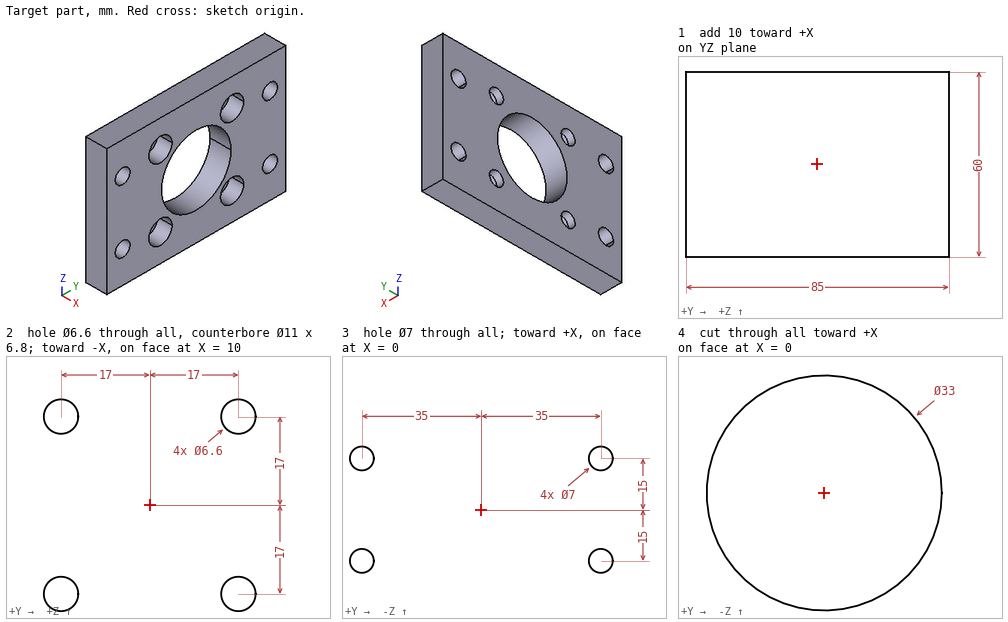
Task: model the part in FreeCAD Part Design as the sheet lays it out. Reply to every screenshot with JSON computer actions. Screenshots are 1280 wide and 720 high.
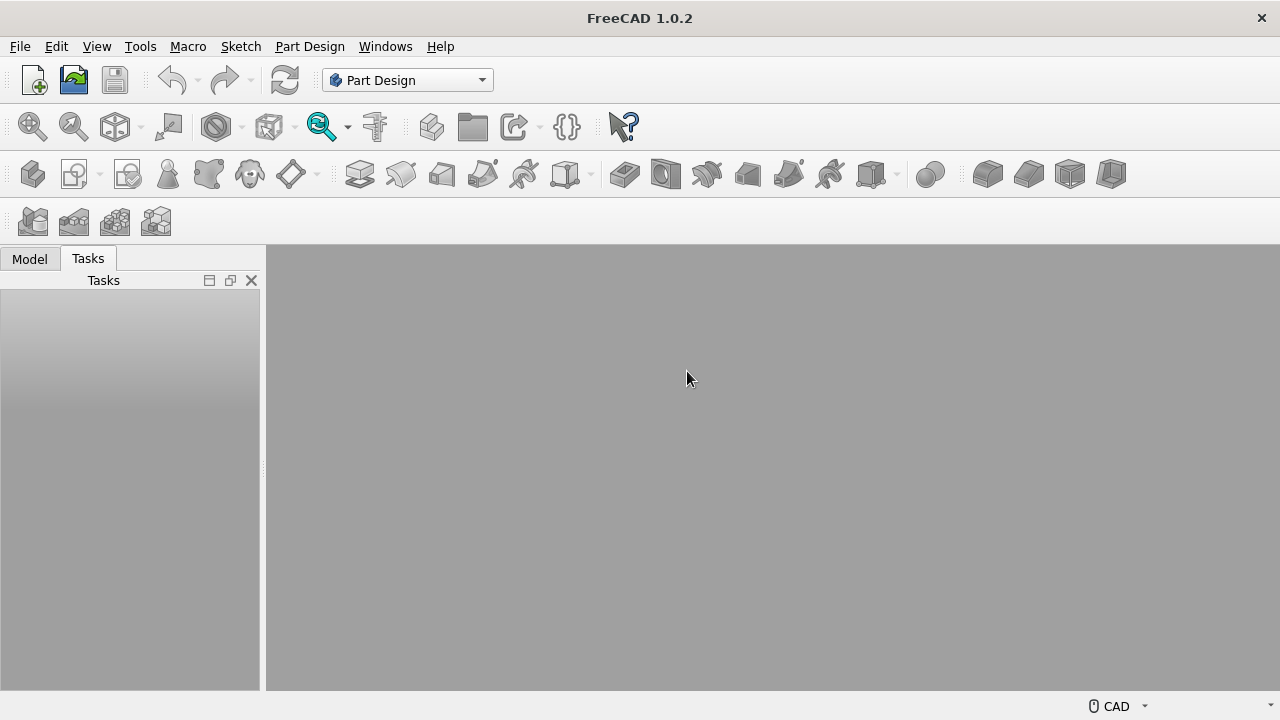
{"action": "left_click", "coordinate": [33, 80]}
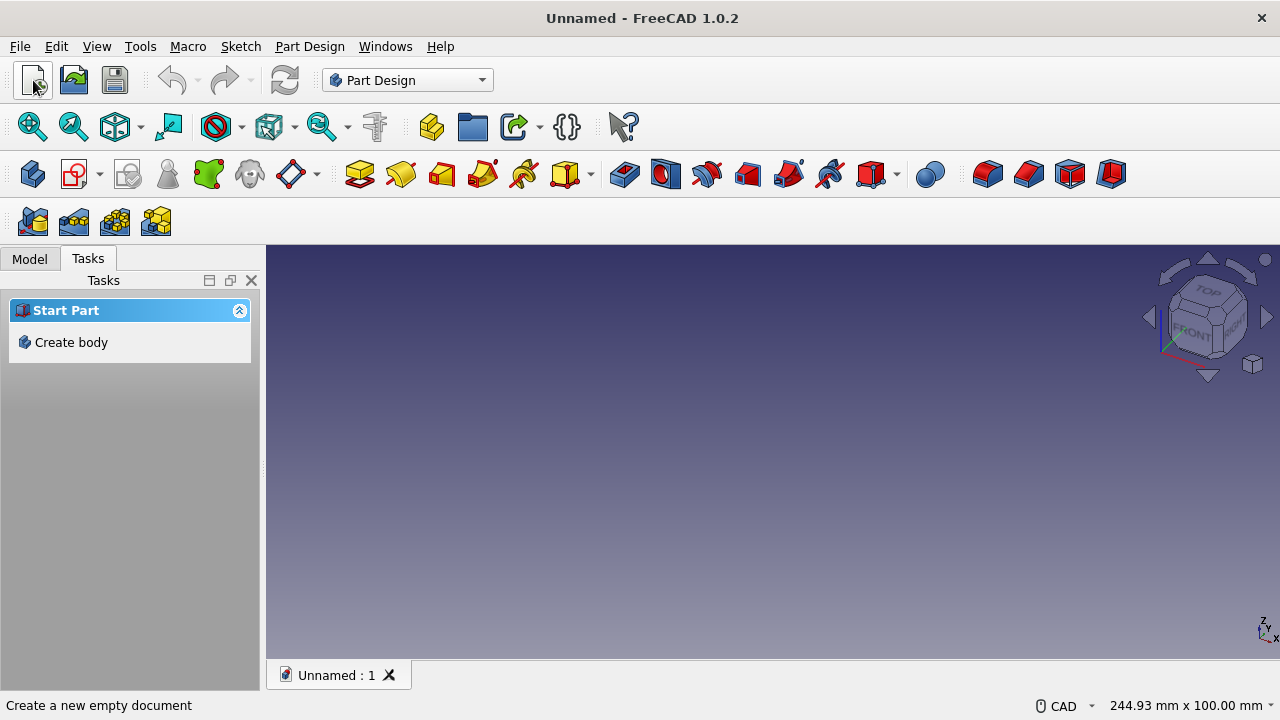
{"action": "left_click", "coordinate": [74, 174]}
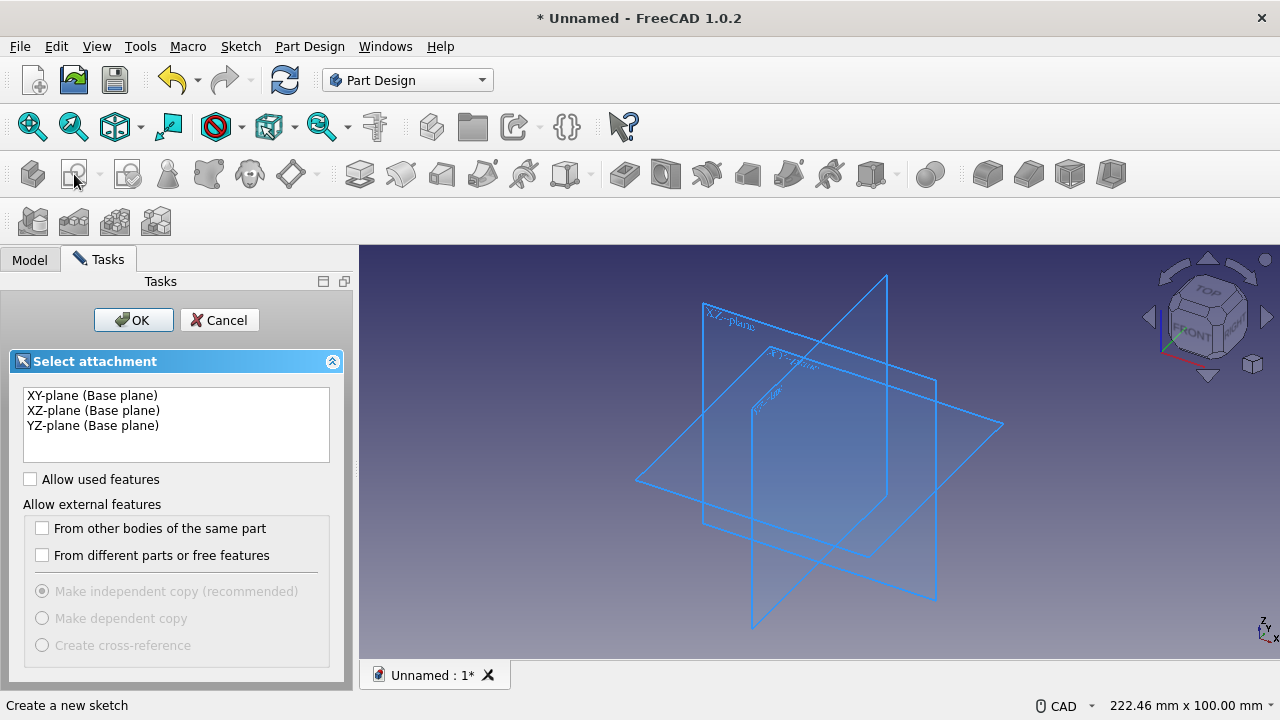
{"action": "left_click", "coordinate": [84, 426]}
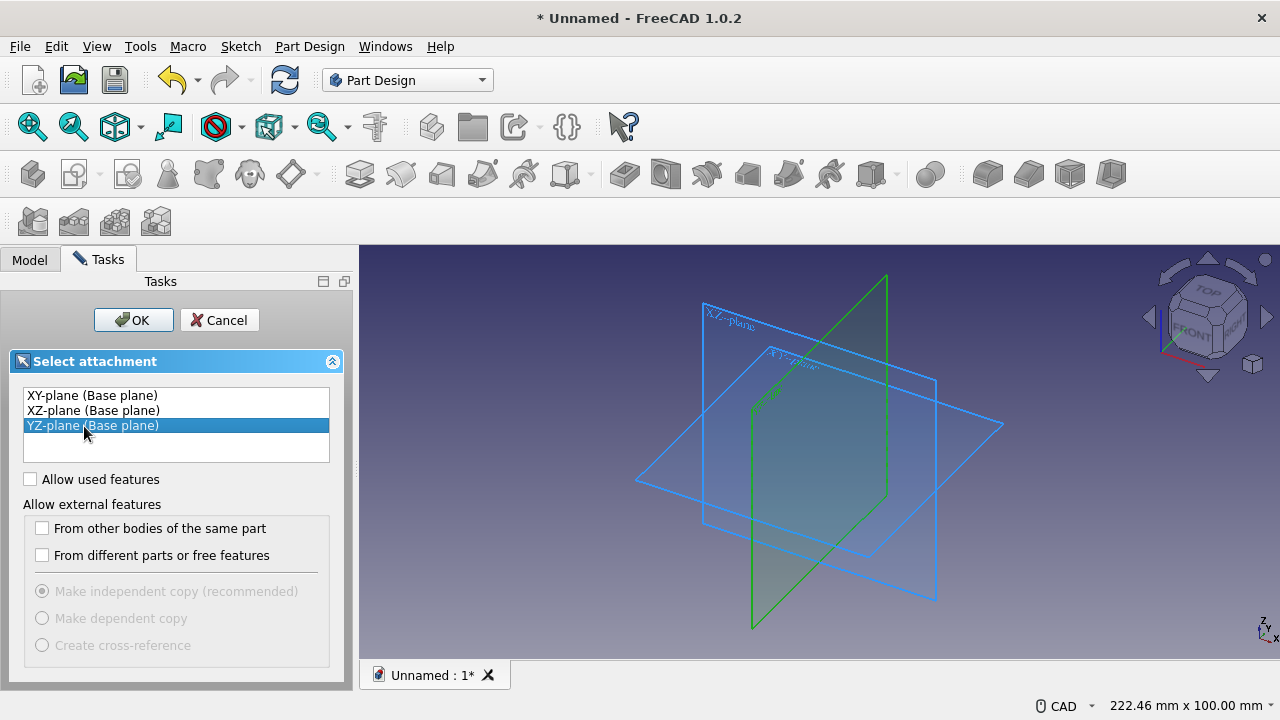
{"action": "left_click", "coordinate": [134, 320]}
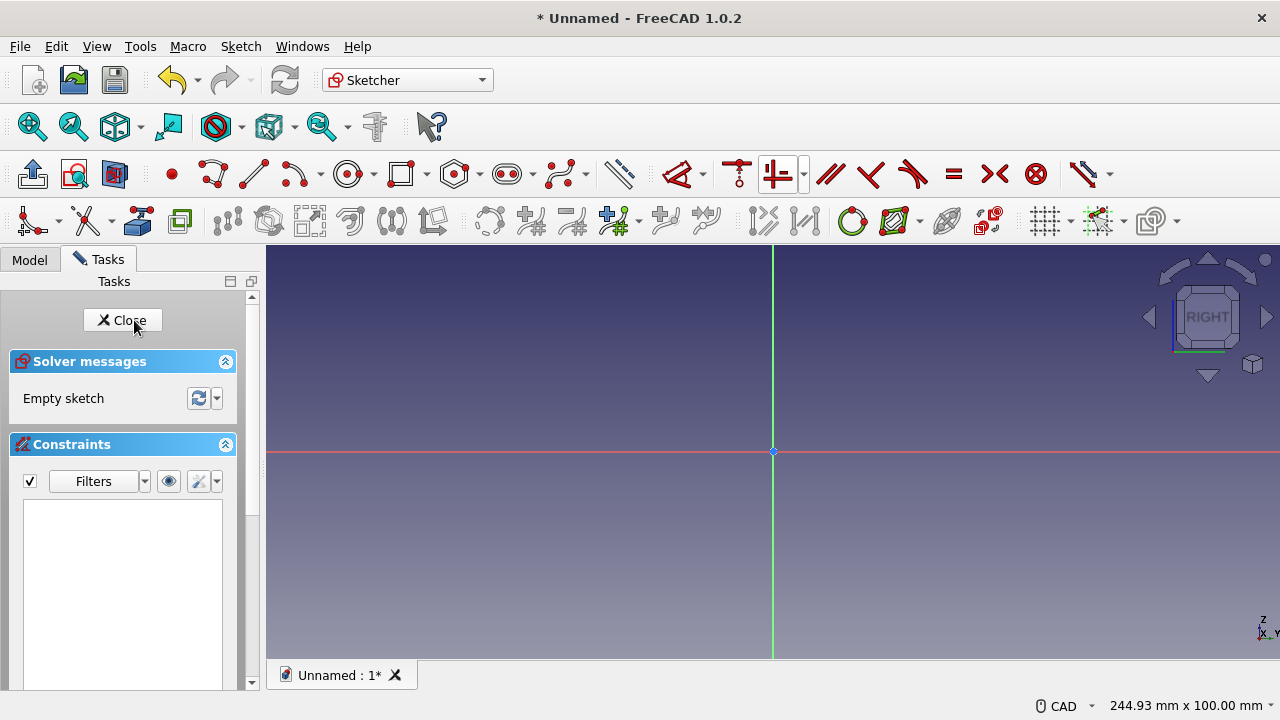
{"action": "key", "text": "g v"}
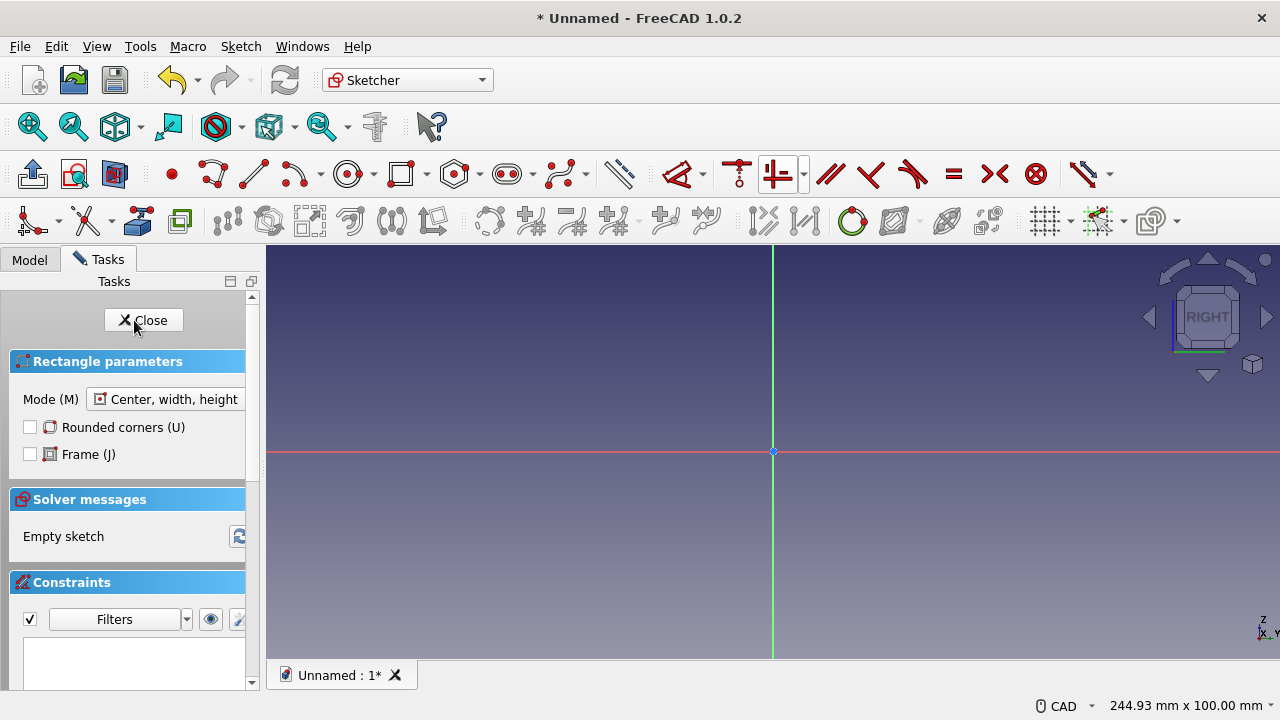
{"action": "left_click", "coordinate": [773, 452]}
{"action": "left_click", "coordinate": [949, 328]}
{"action": "key", "text": "Escape"}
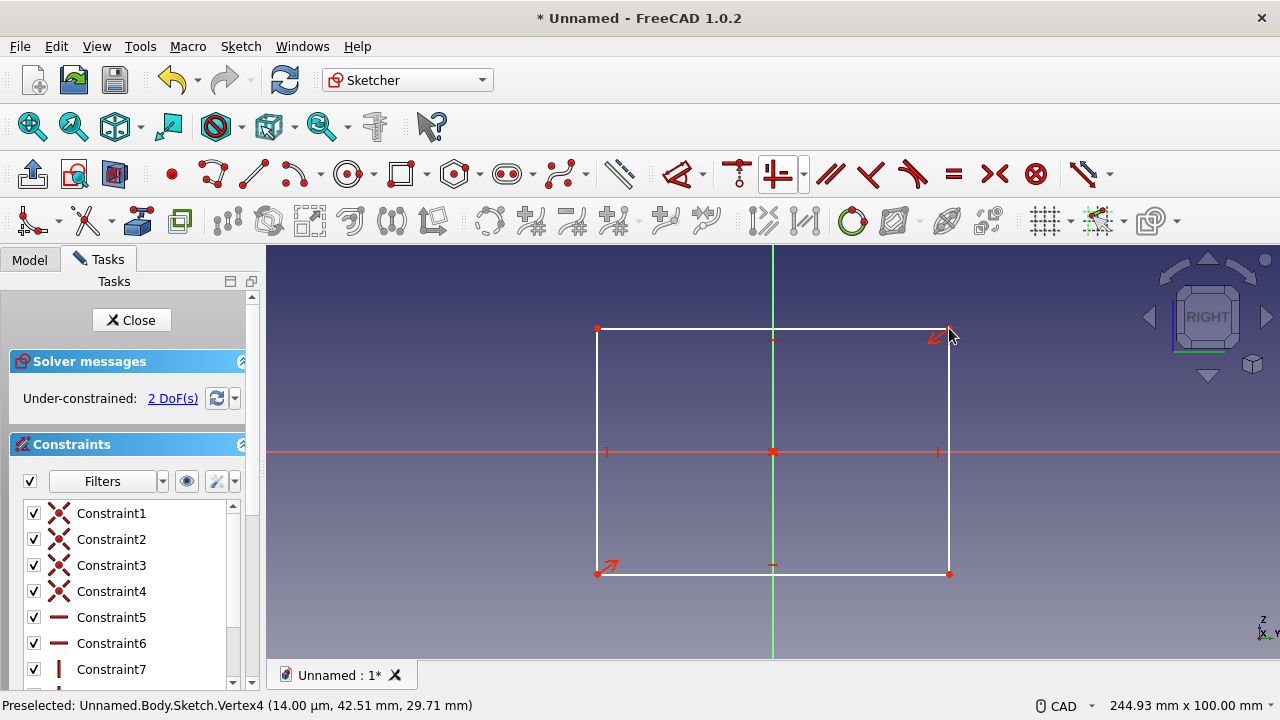
{"action": "left_click", "coordinate": [703, 575]}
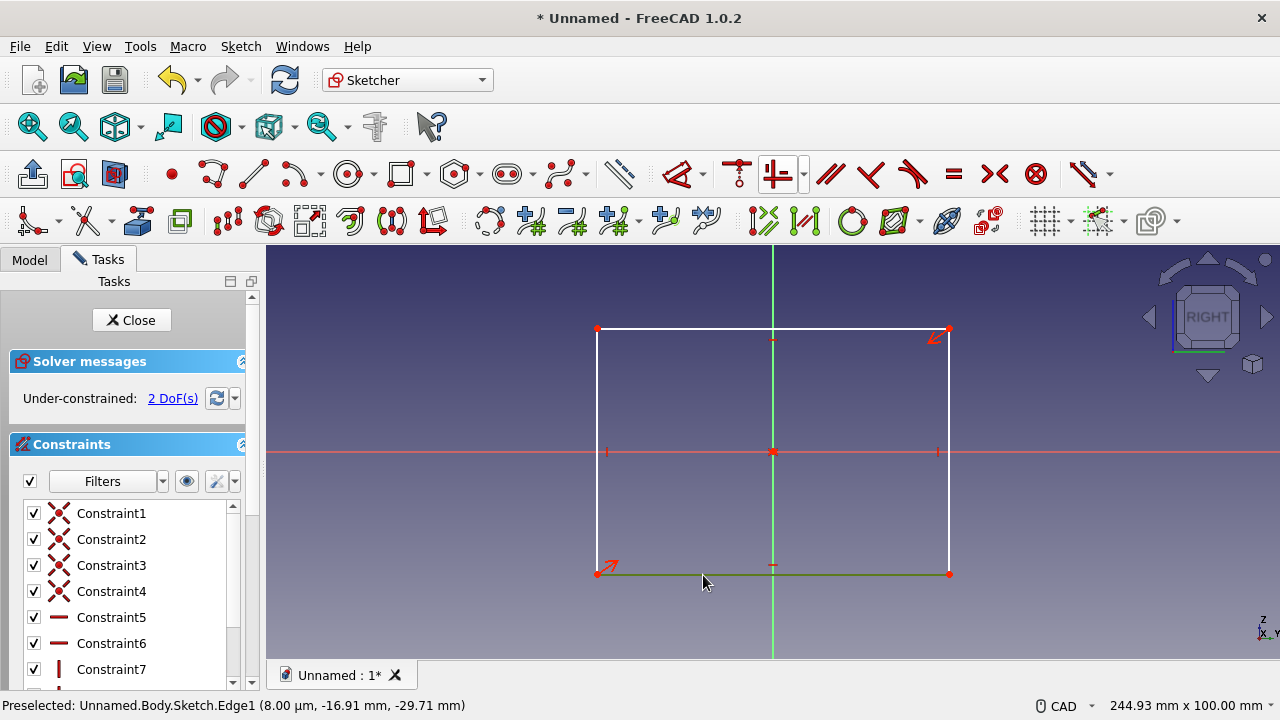
{"action": "key", "text": "l"}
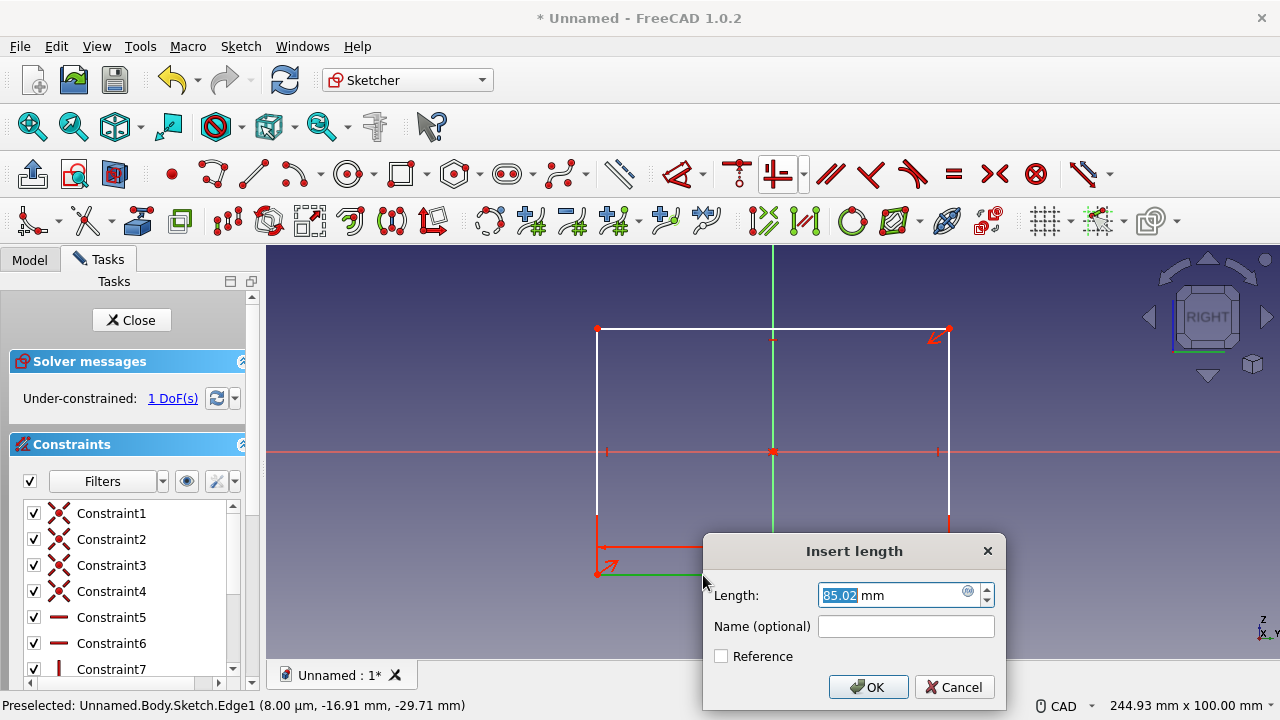
{"action": "type", "text": "85"}
{"action": "key", "text": "Return"}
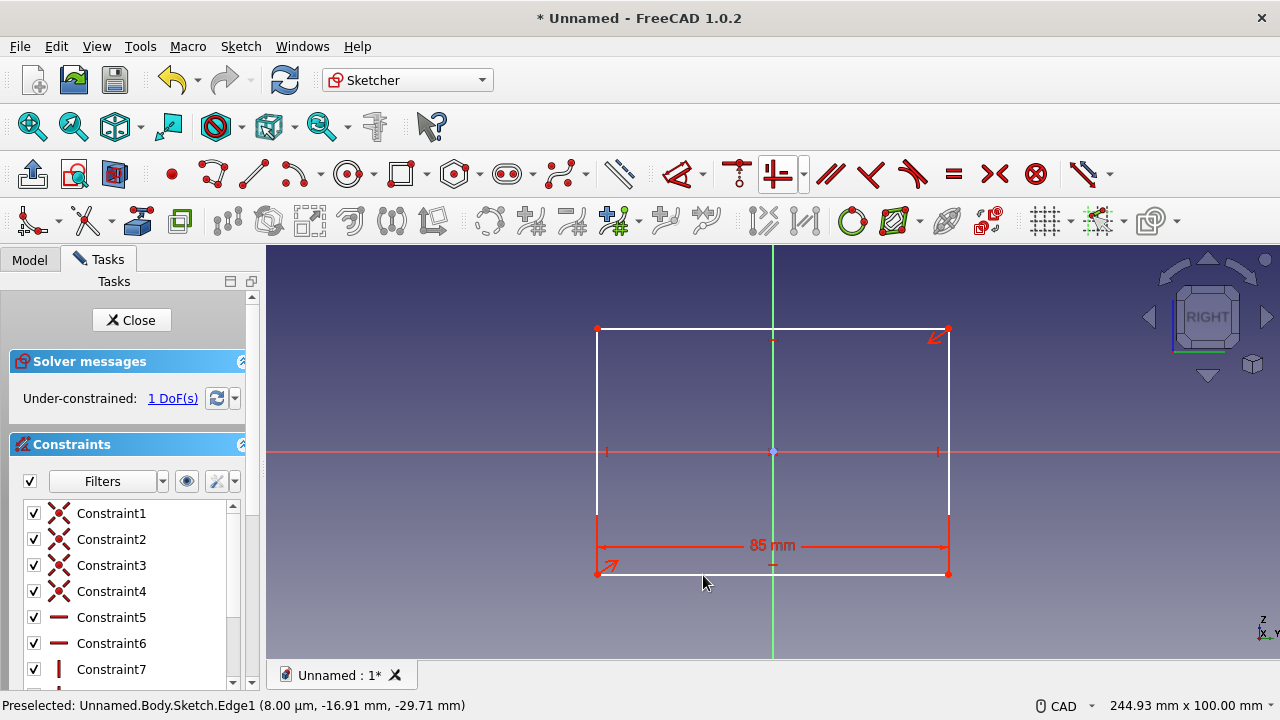
{"action": "left_click", "coordinate": [949, 501]}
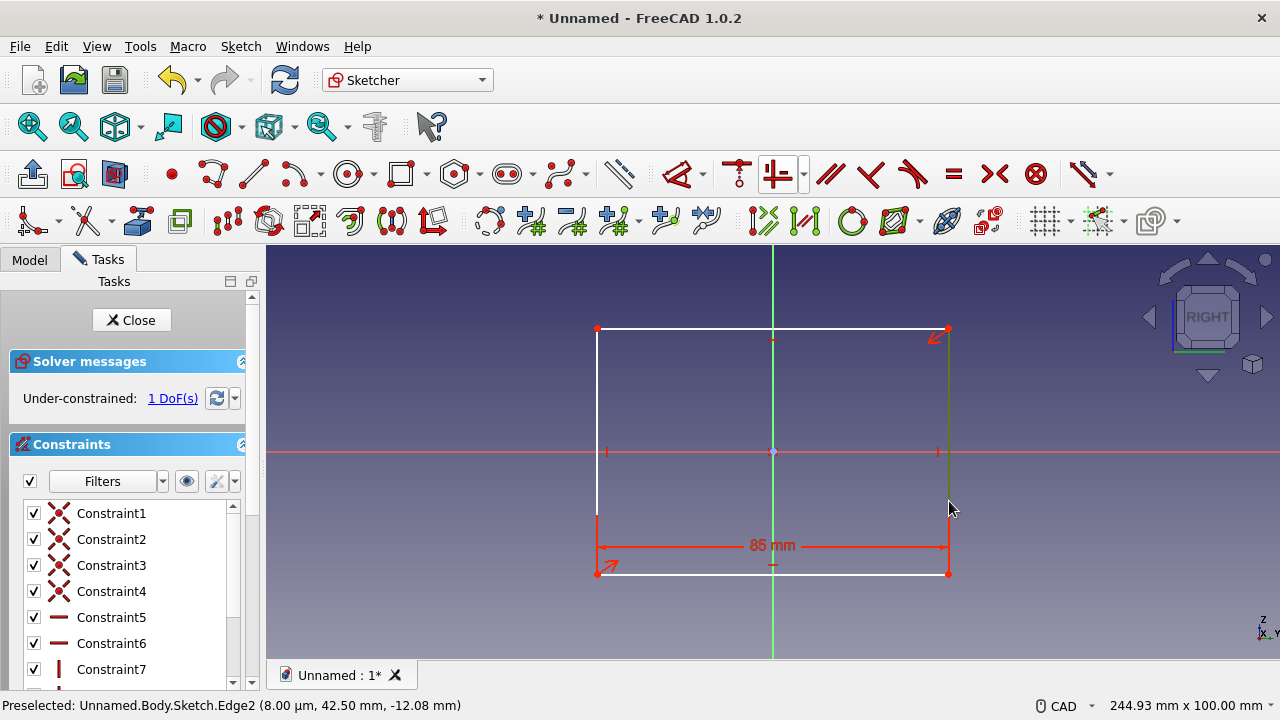
{"action": "key", "text": "i"}